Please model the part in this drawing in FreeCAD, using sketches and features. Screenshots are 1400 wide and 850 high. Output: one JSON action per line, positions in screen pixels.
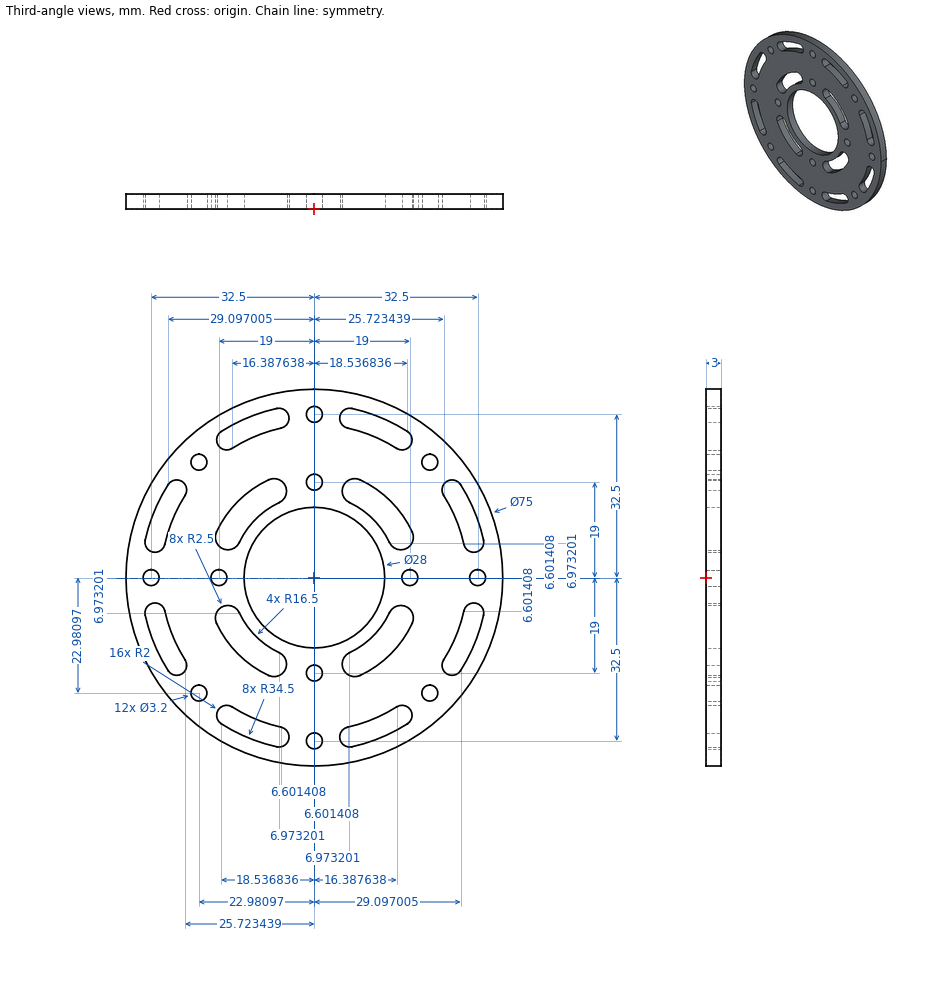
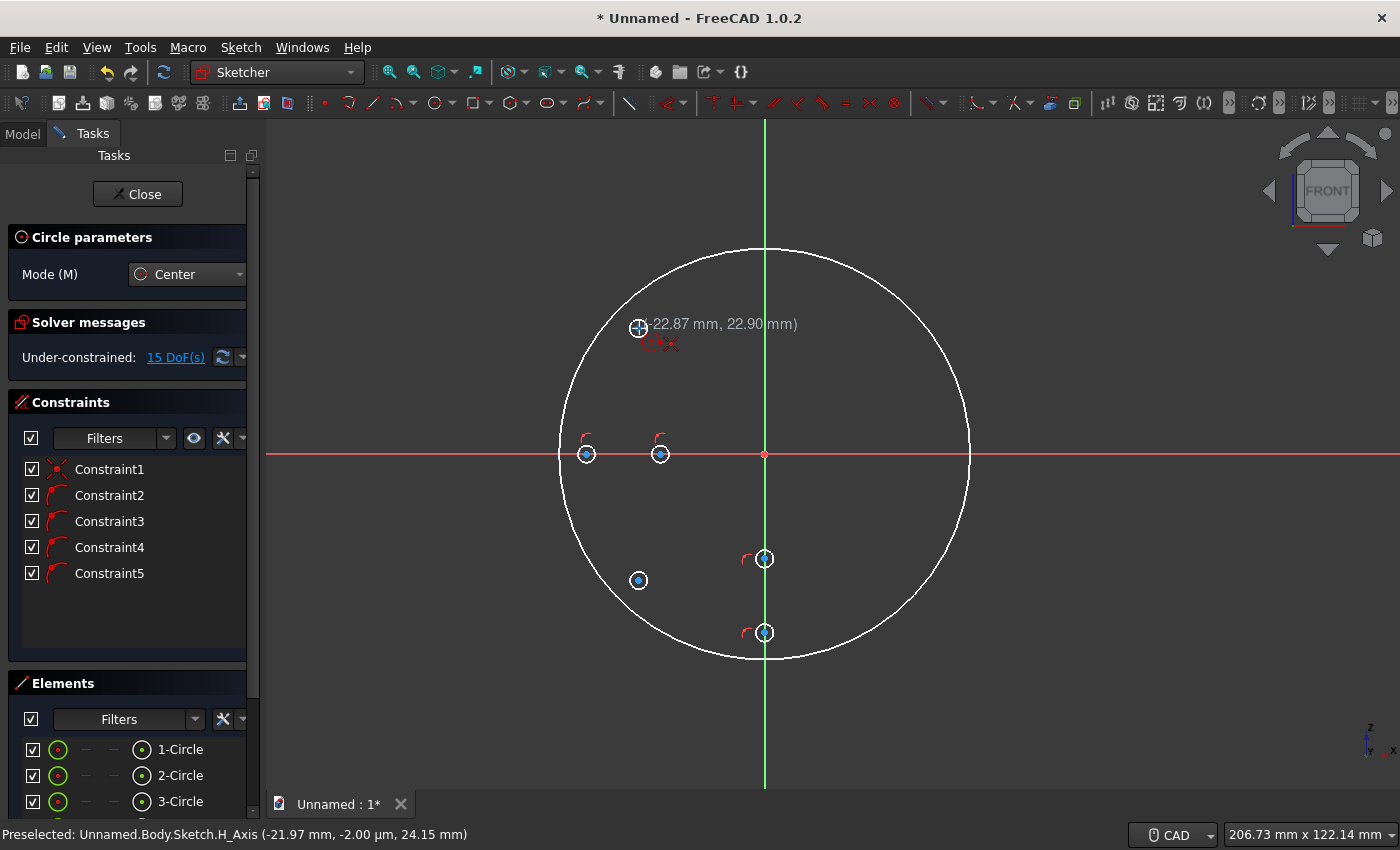
{"action": "scroll", "coordinate": [891, 580], "scroll_direction": "up", "scroll_amount": 5}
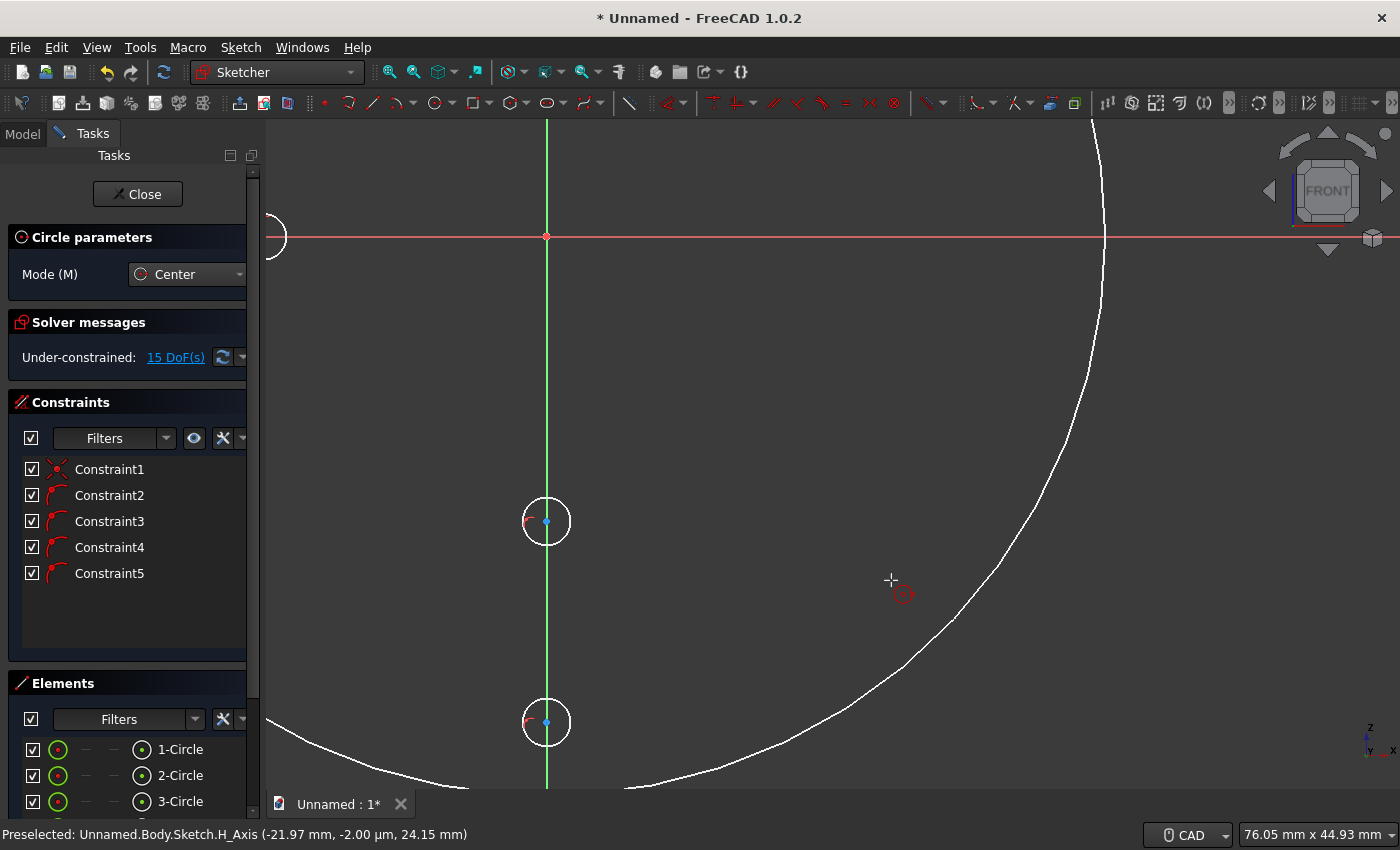
{"action": "left_click", "coordinate": [889, 580]}
{"action": "left_click", "coordinate": [906, 563]}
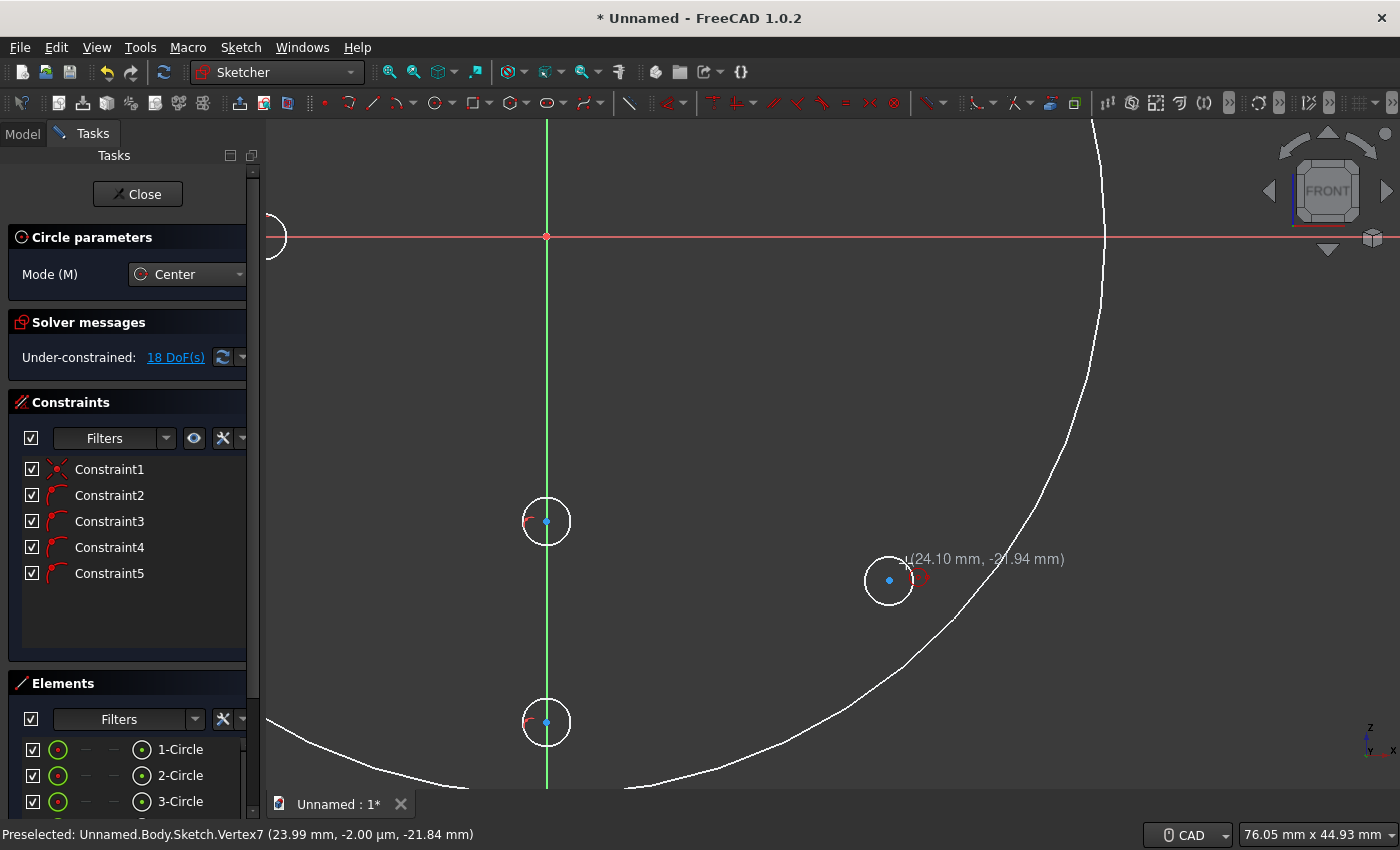
{"action": "left_click", "coordinate": [1031, 237]}
{"action": "left_click", "coordinate": [1048, 220]}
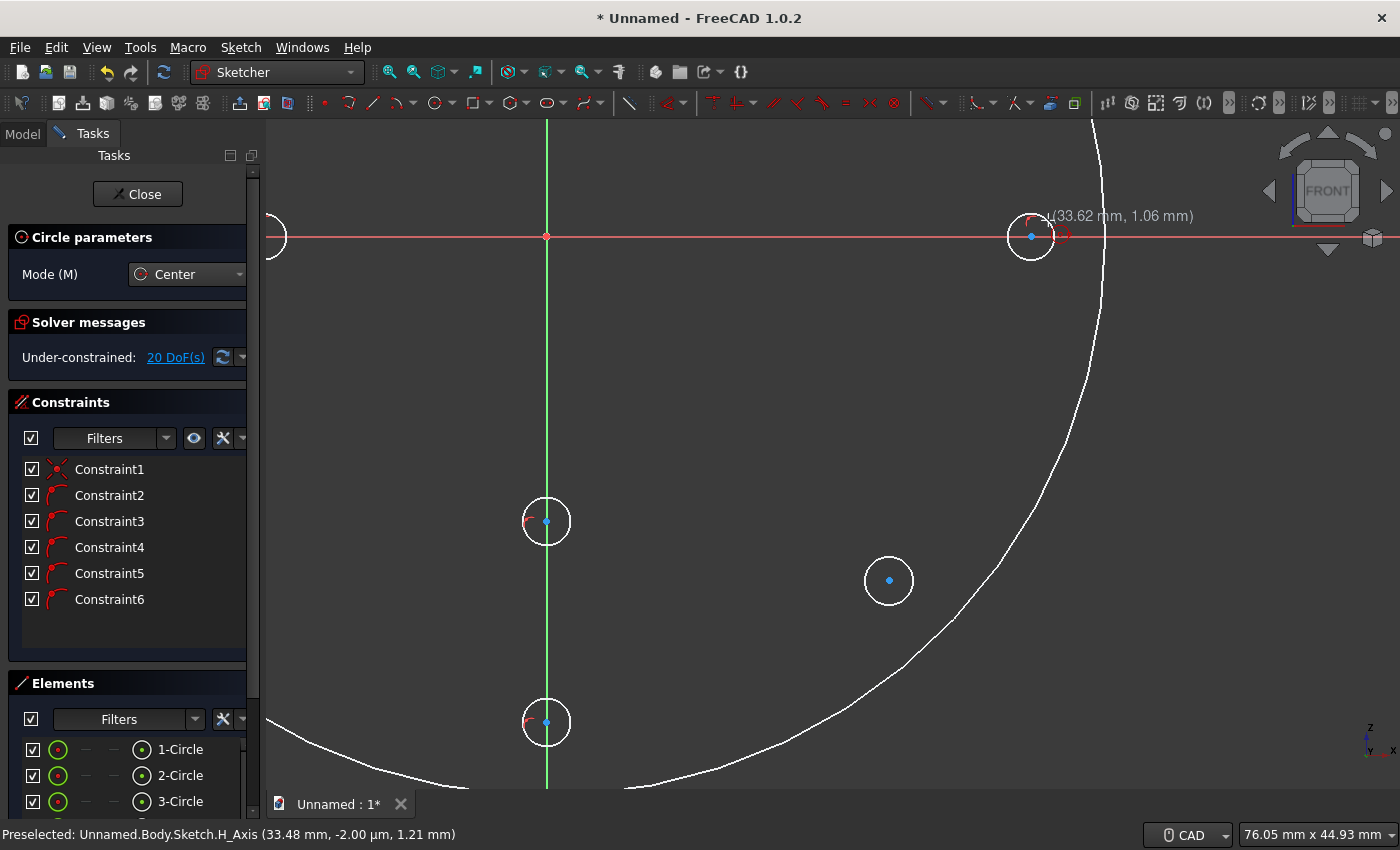
{"action": "left_click", "coordinate": [547, 237]}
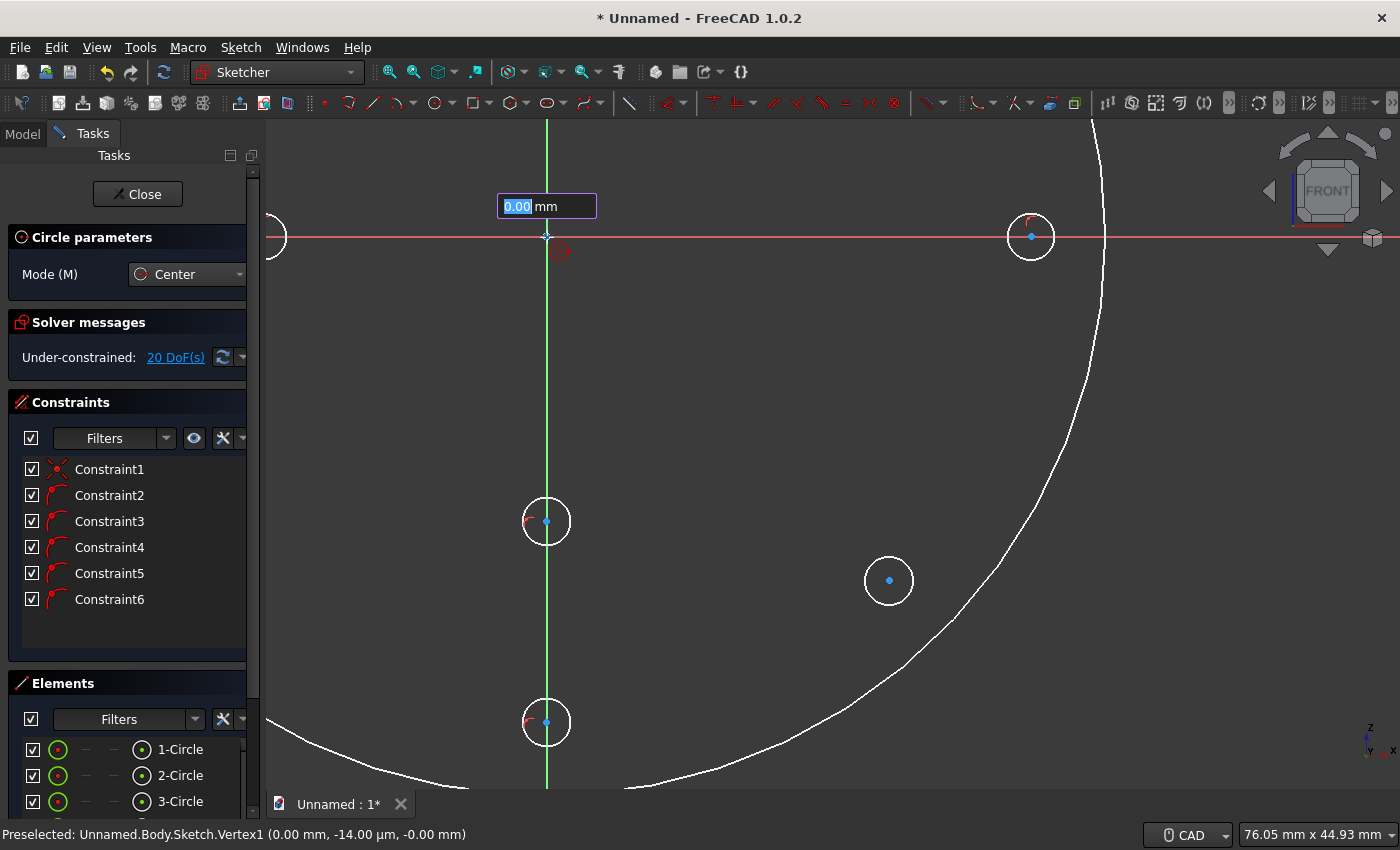
{"action": "scroll", "coordinate": [891, 580], "scroll_direction": "down", "scroll_amount": 5}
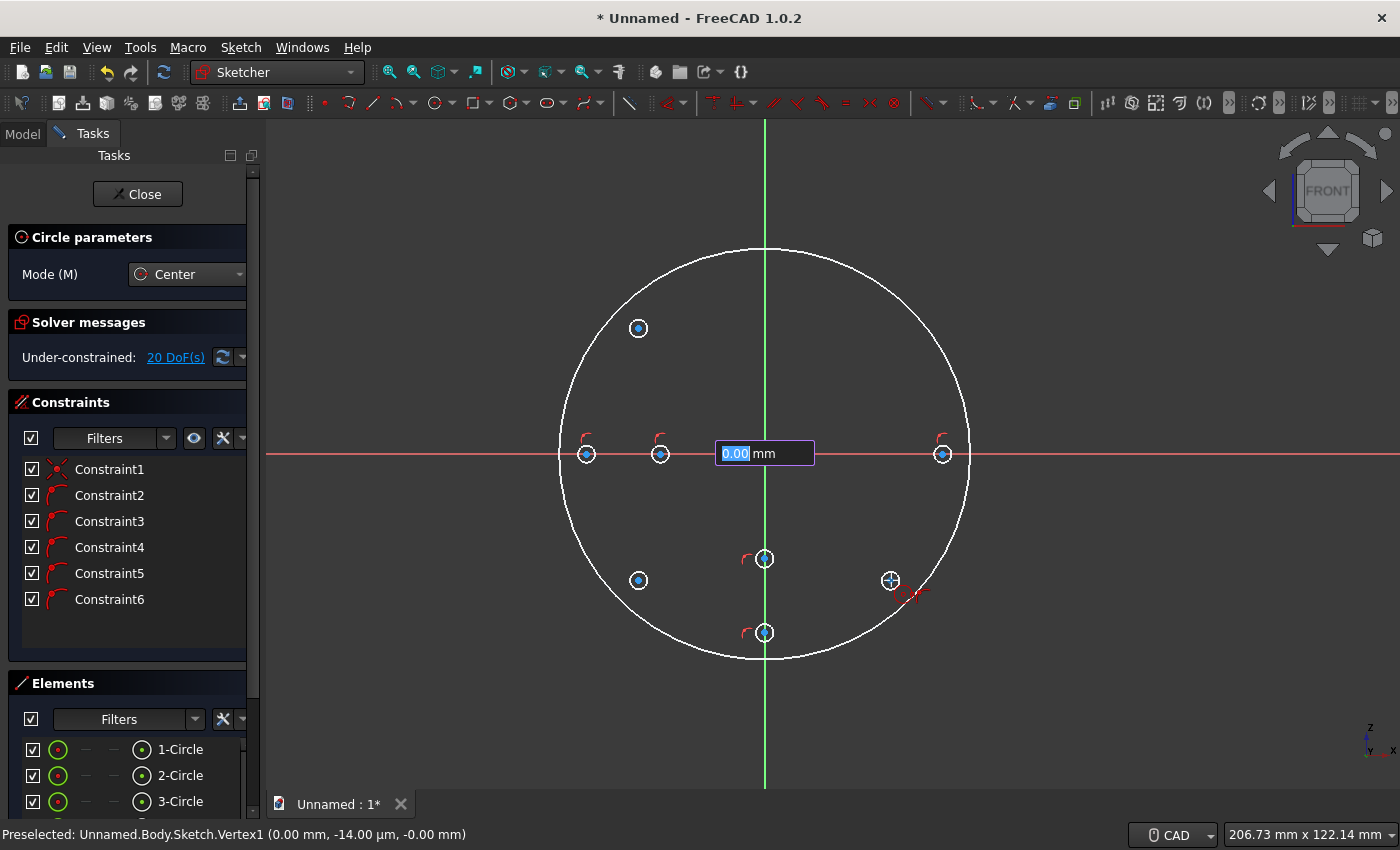
{"action": "left_click", "coordinate": [819, 400]}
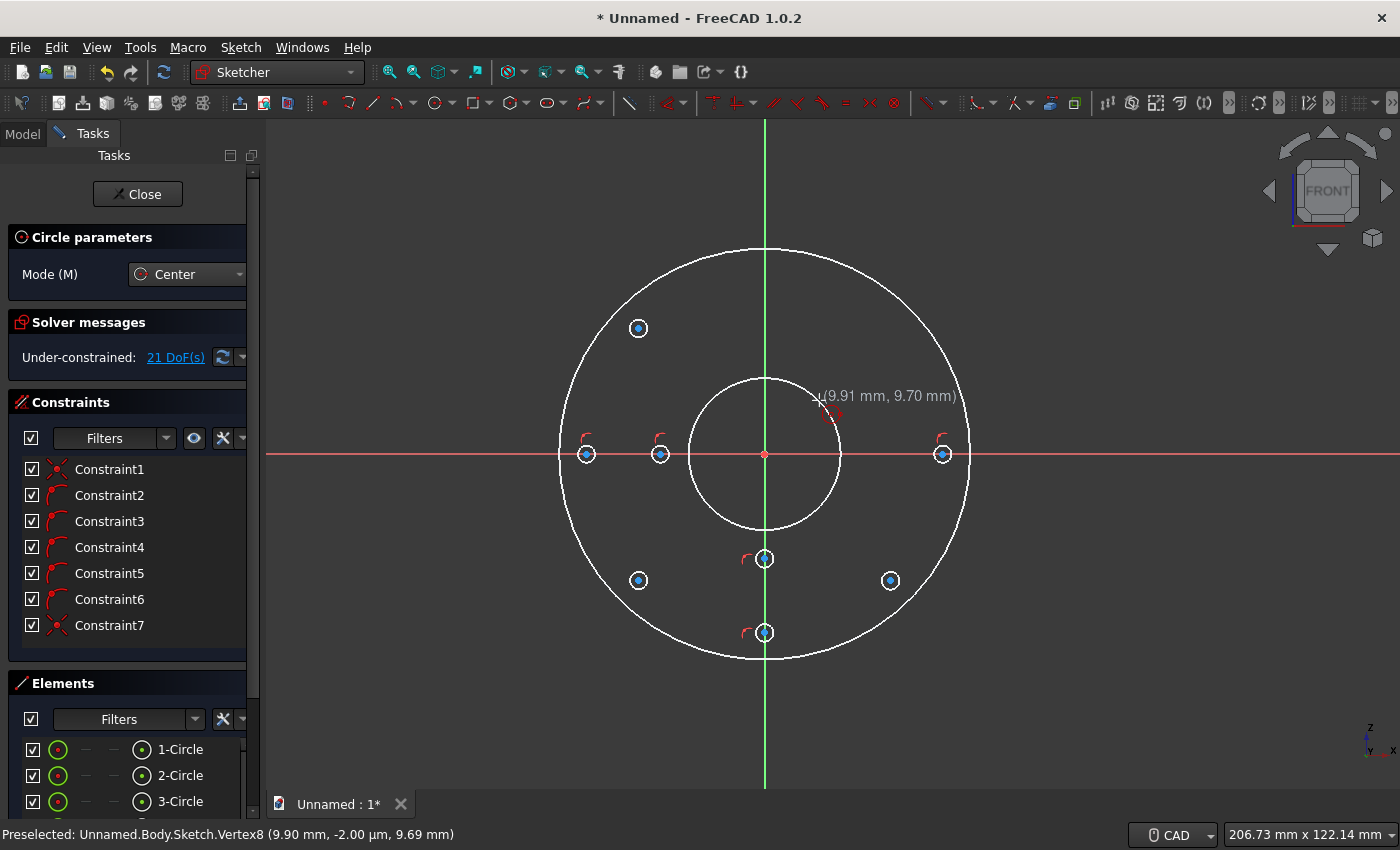
{"action": "scroll", "coordinate": [765, 350], "scroll_direction": "up", "scroll_amount": 5}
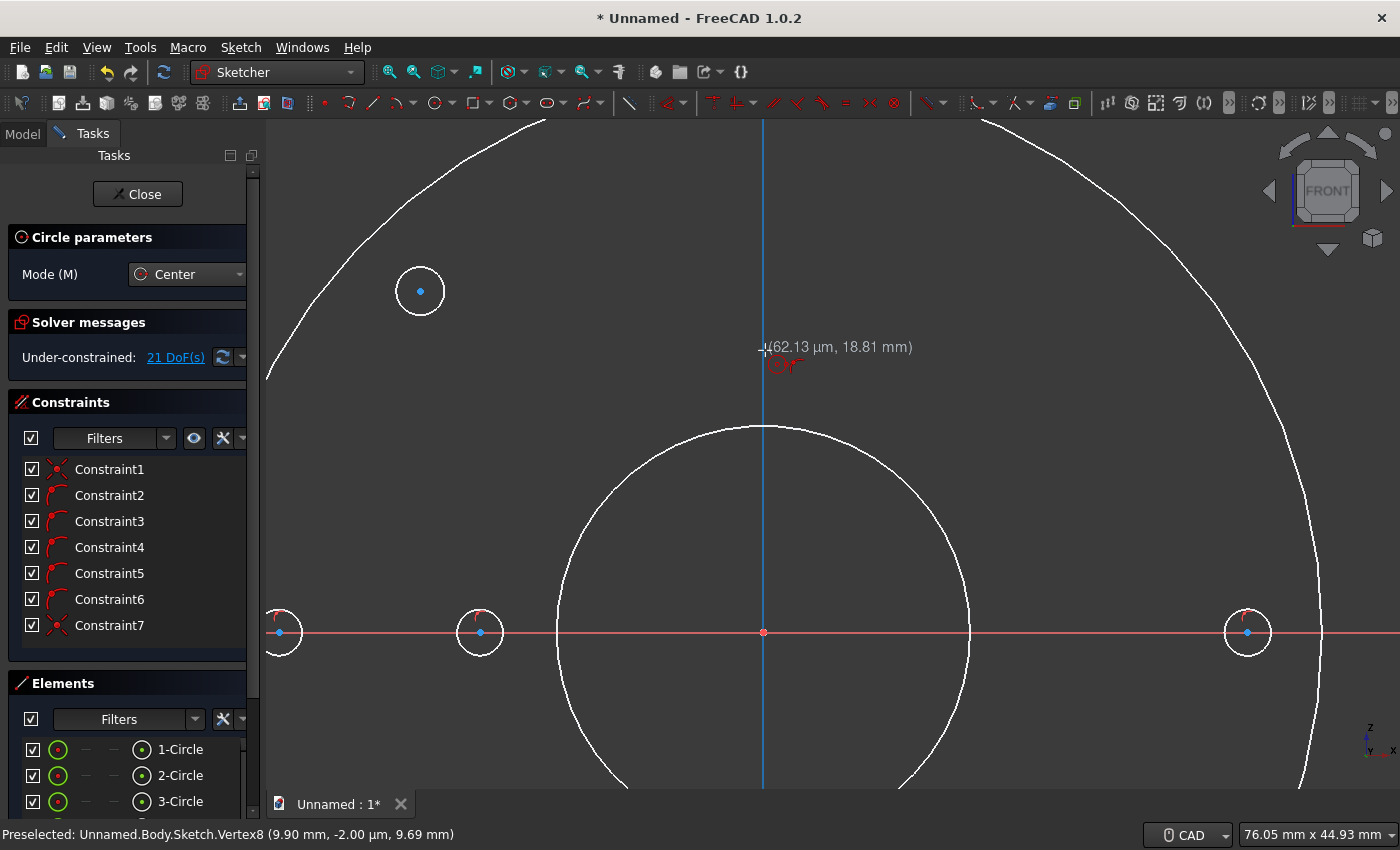
{"action": "left_click", "coordinate": [763, 349]}
{"action": "left_click", "coordinate": [780, 332]}